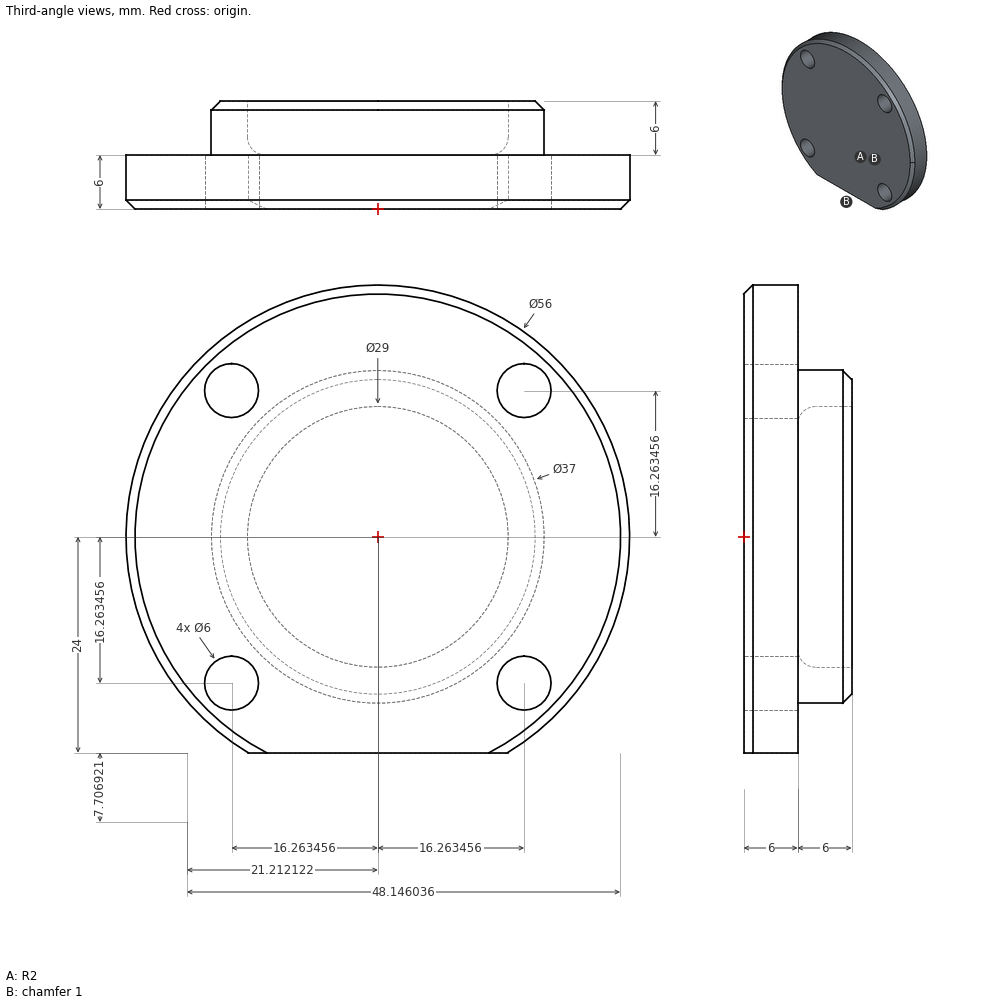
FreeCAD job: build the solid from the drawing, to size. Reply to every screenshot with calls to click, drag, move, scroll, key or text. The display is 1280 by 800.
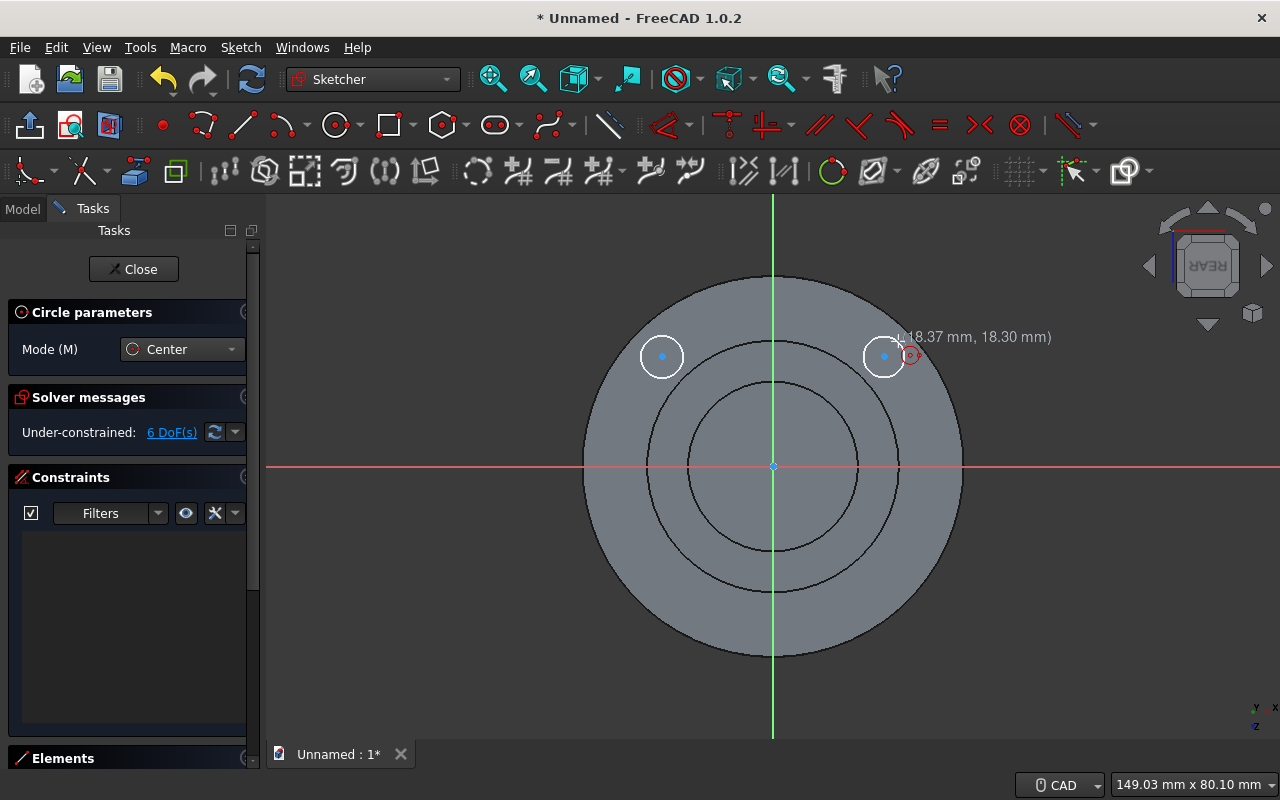
click(884, 577)
click(898, 563)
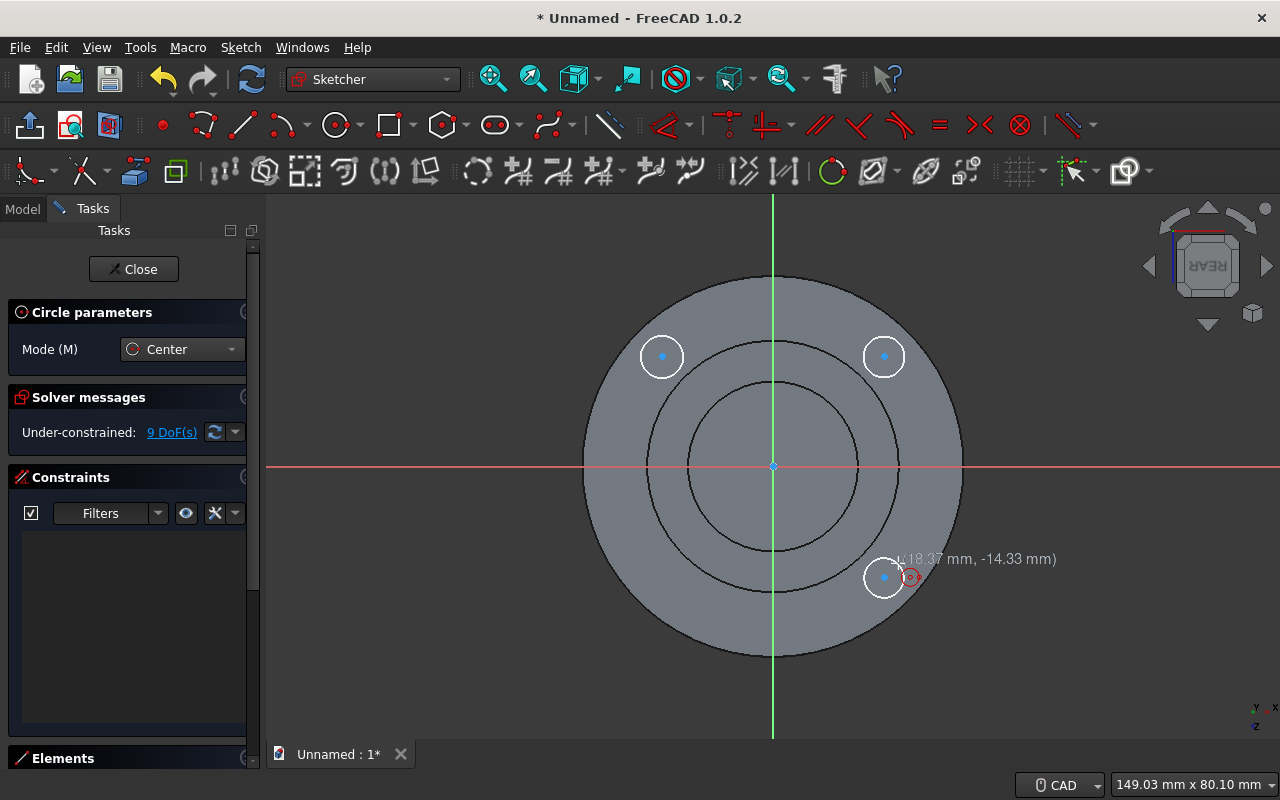
click(662, 577)
click(677, 563)
key(Escape)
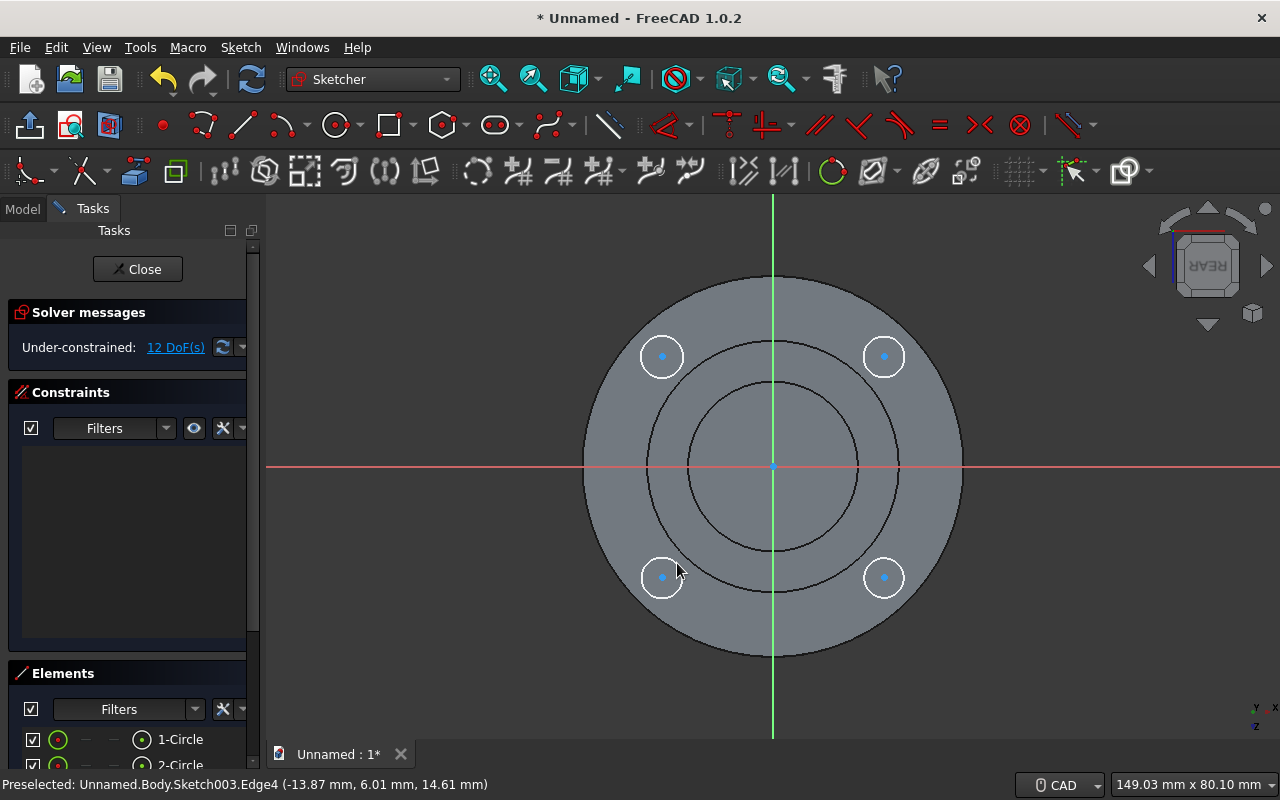
click(677, 342)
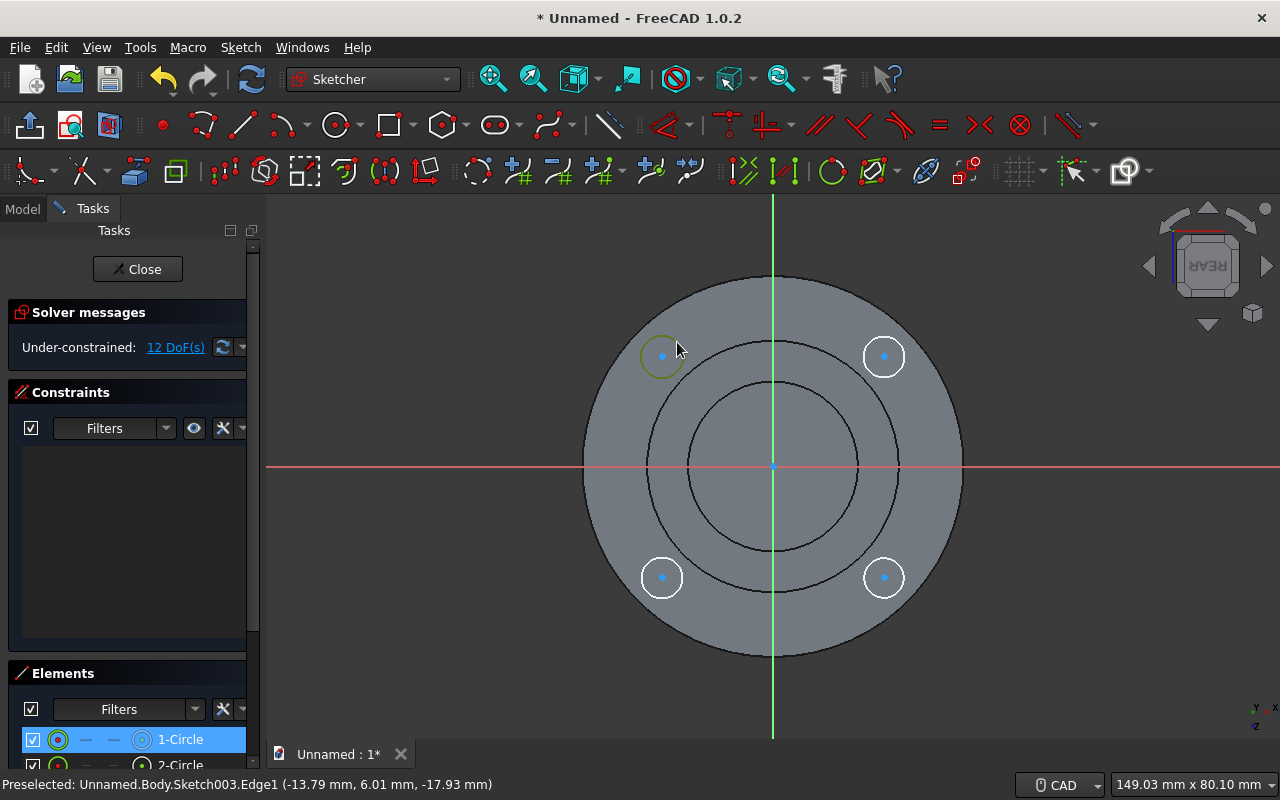
click(898, 342)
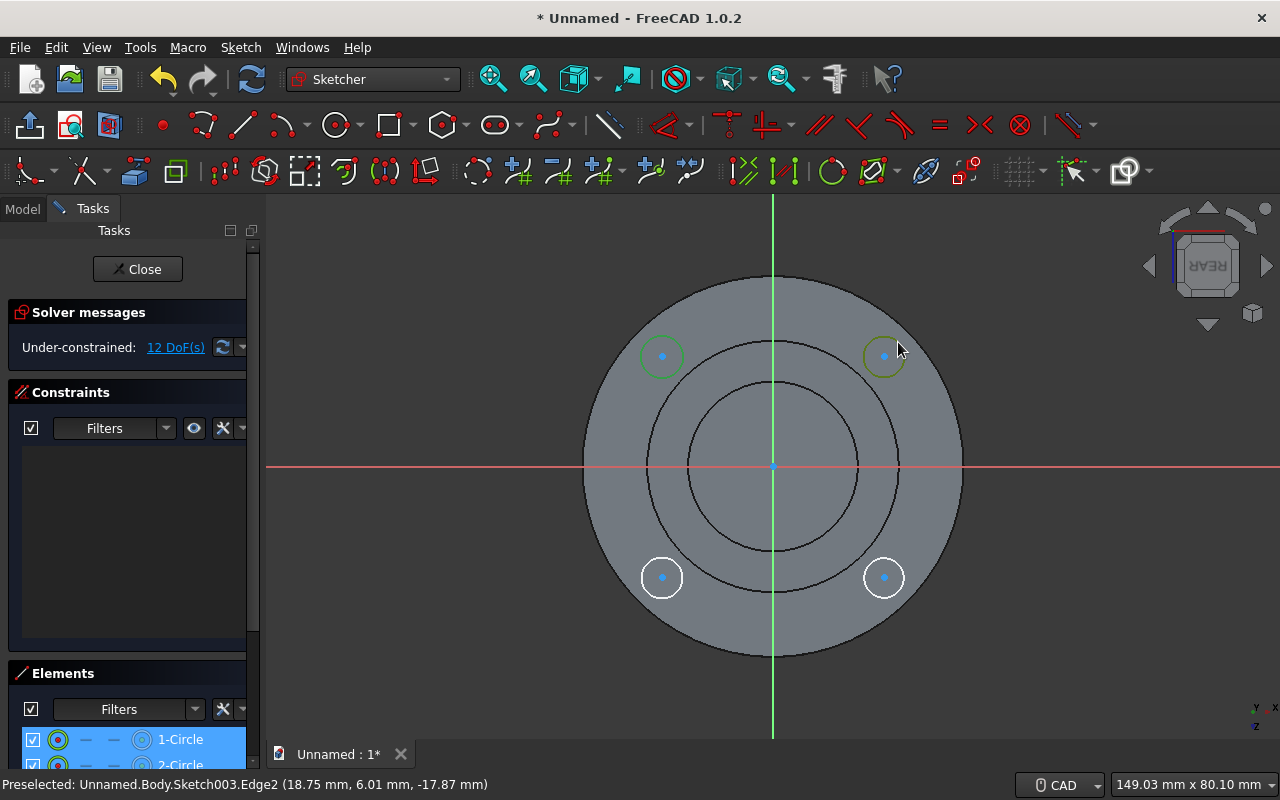
click(898, 564)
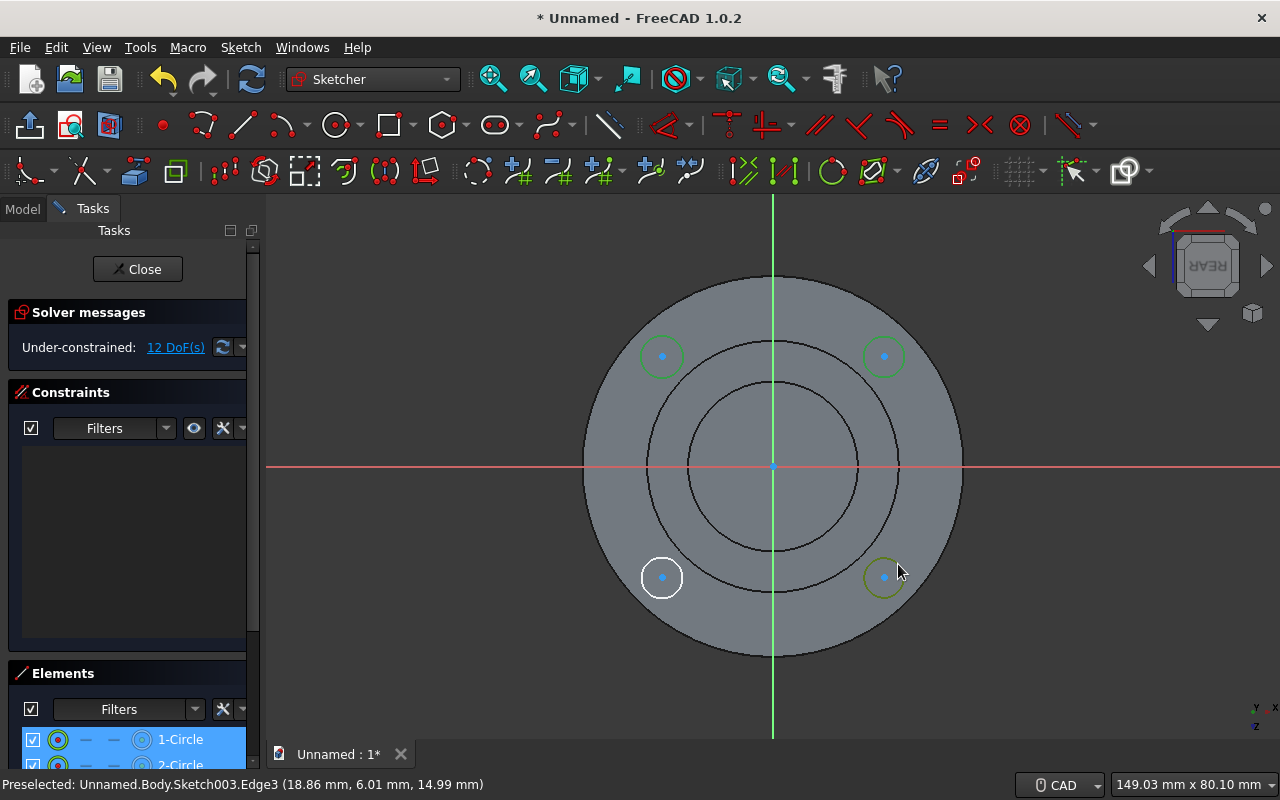
click(676, 563)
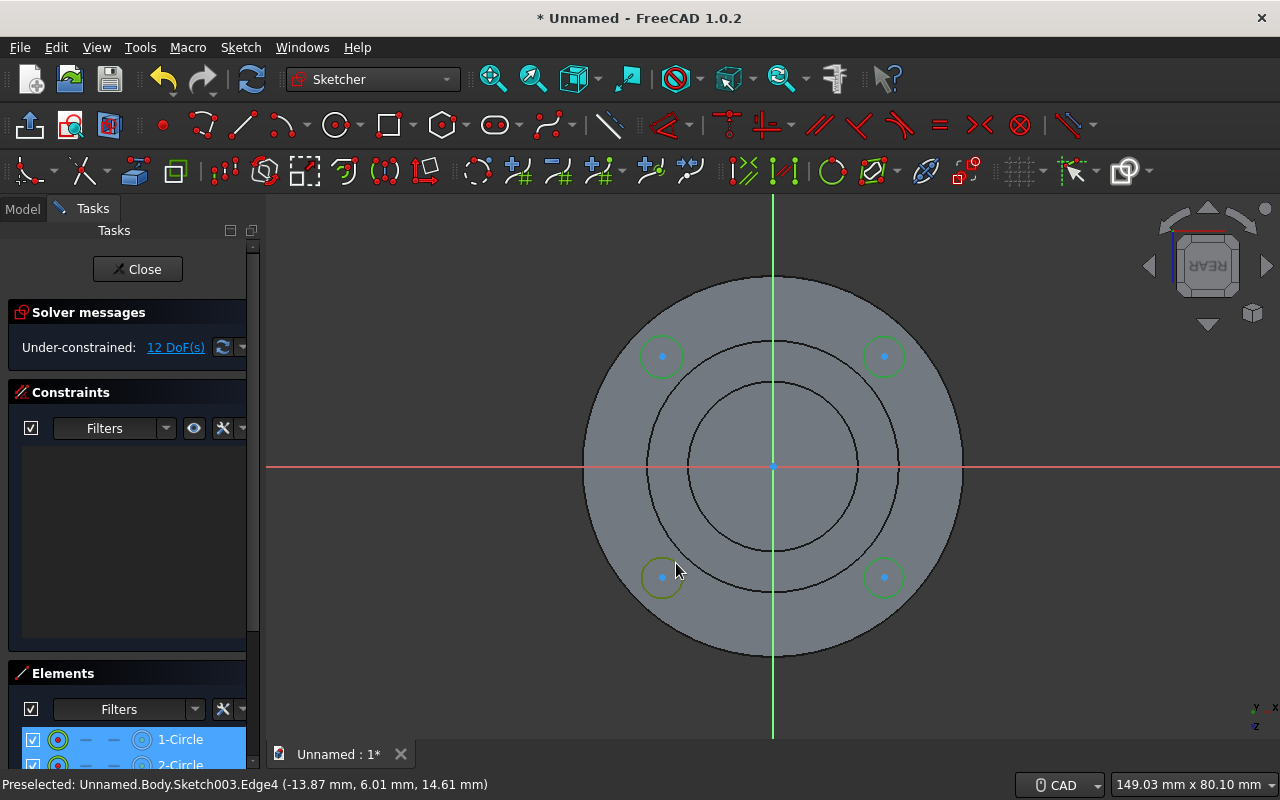
key(e)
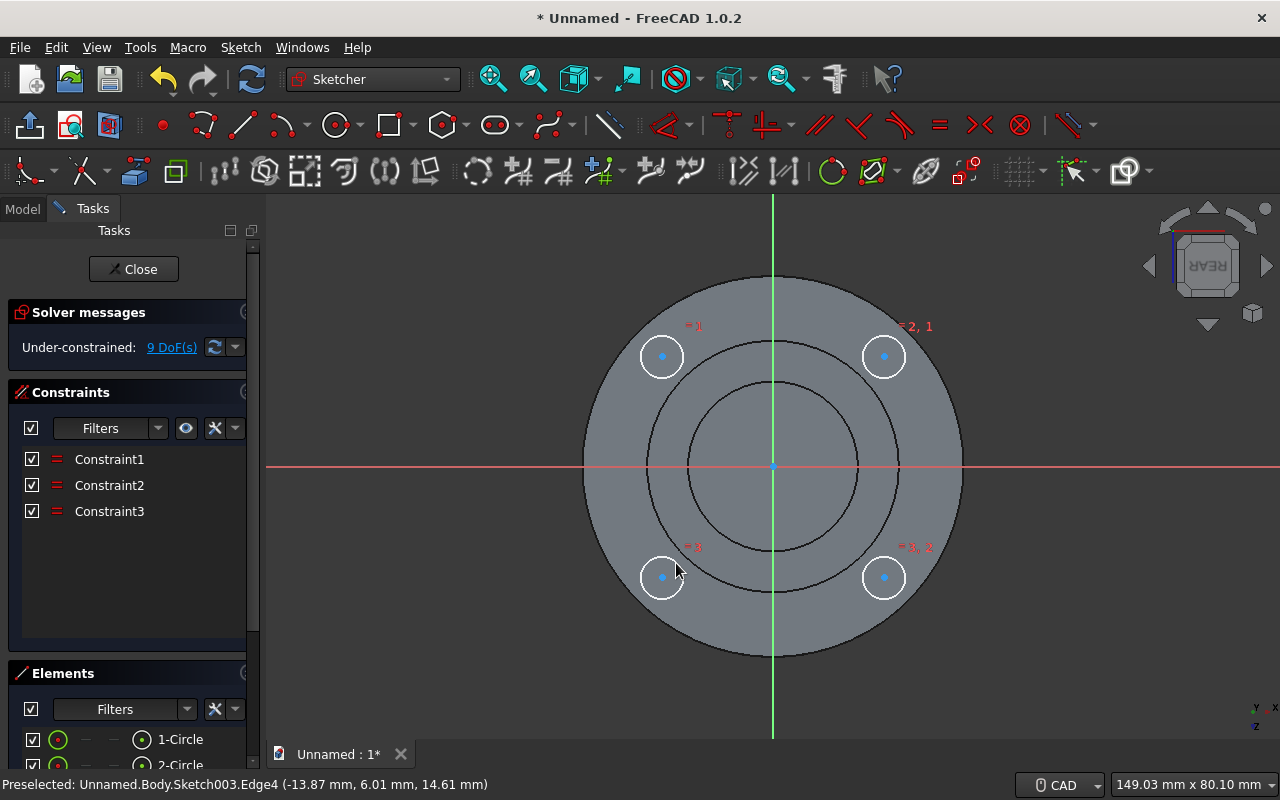
click(662, 357)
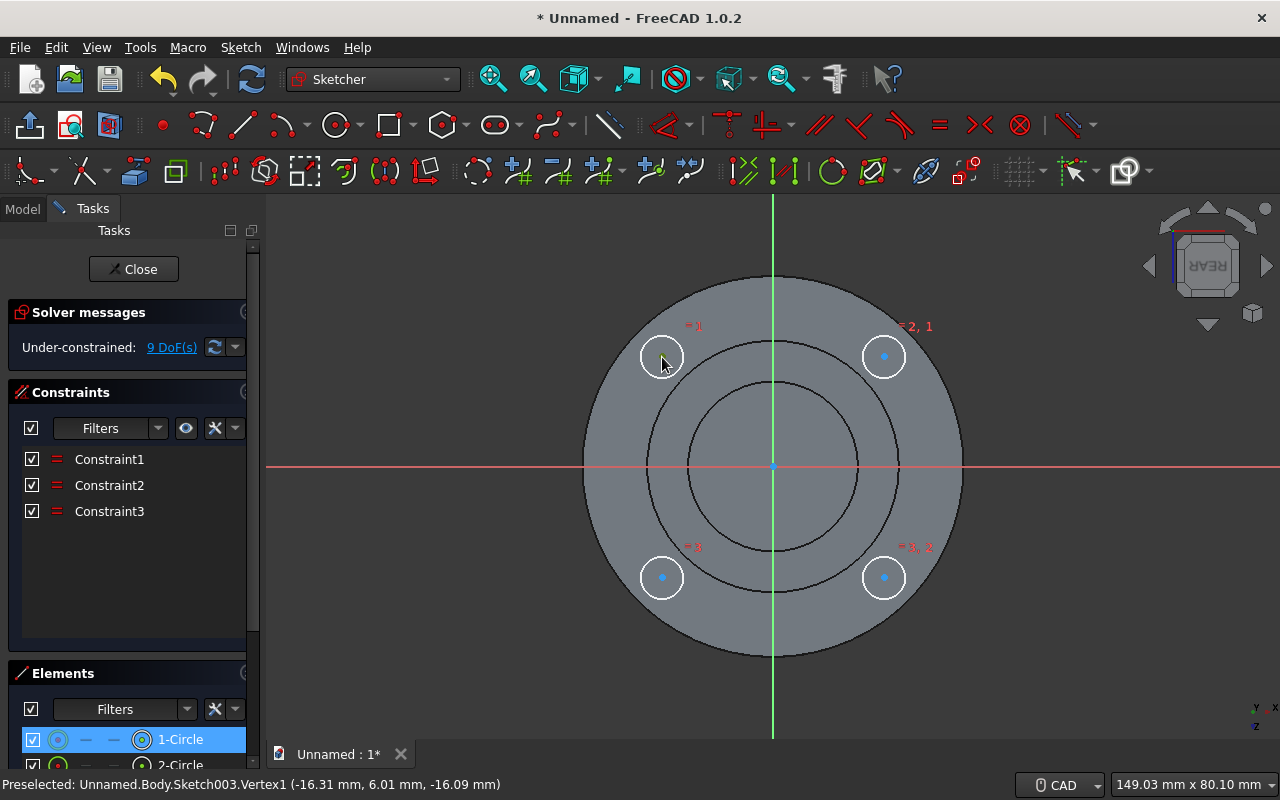
click(884, 357)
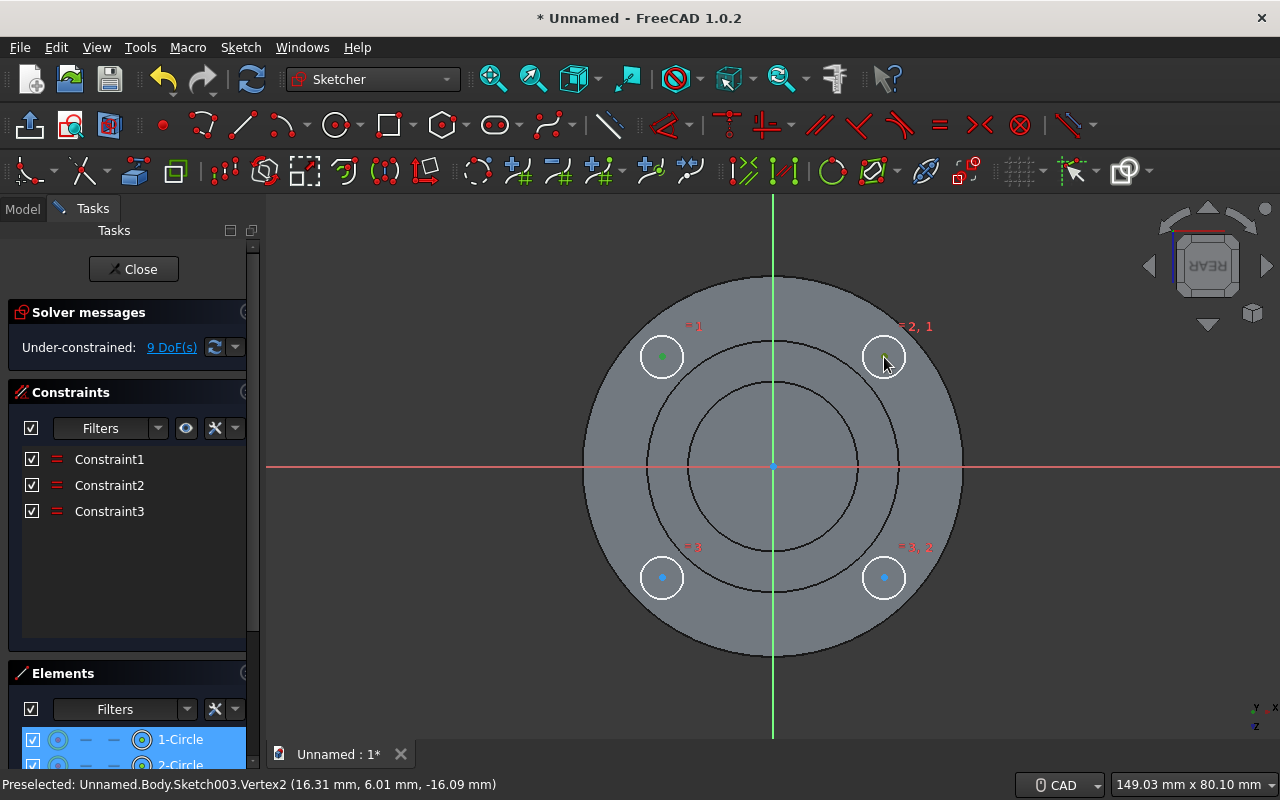
key(h)